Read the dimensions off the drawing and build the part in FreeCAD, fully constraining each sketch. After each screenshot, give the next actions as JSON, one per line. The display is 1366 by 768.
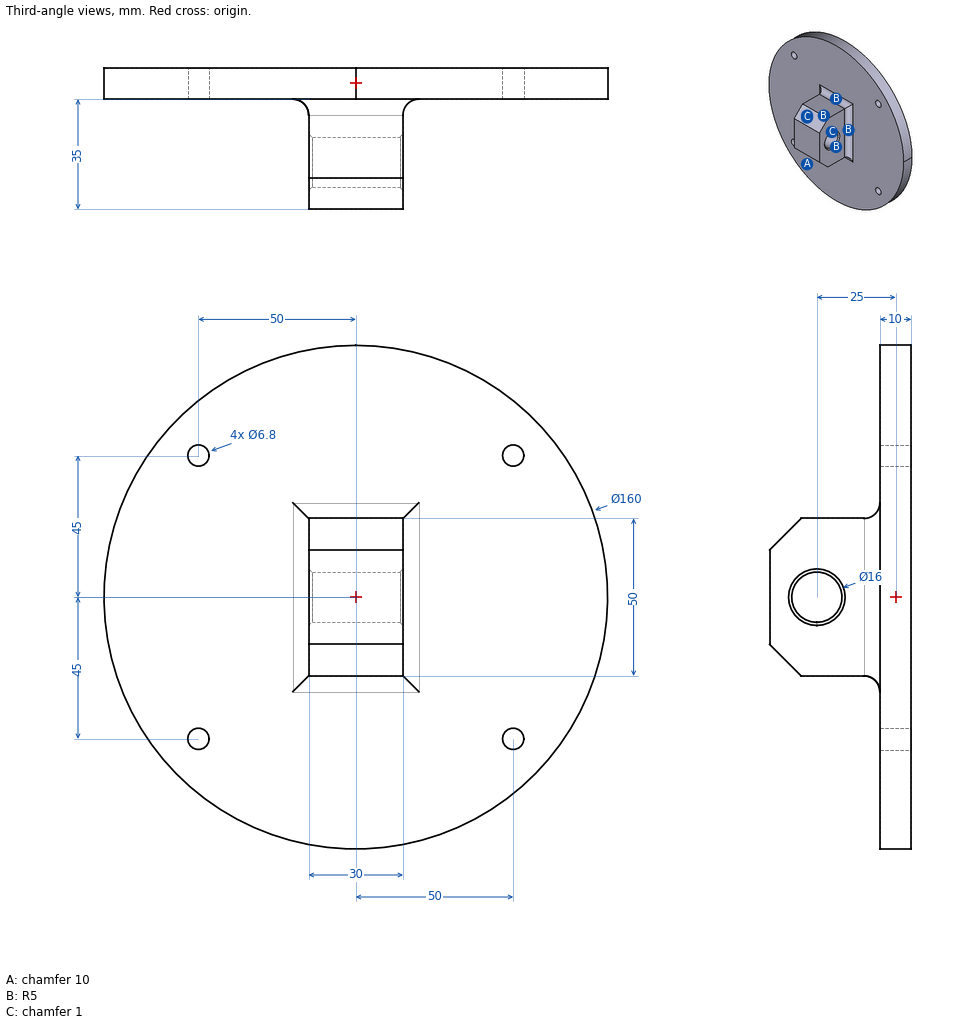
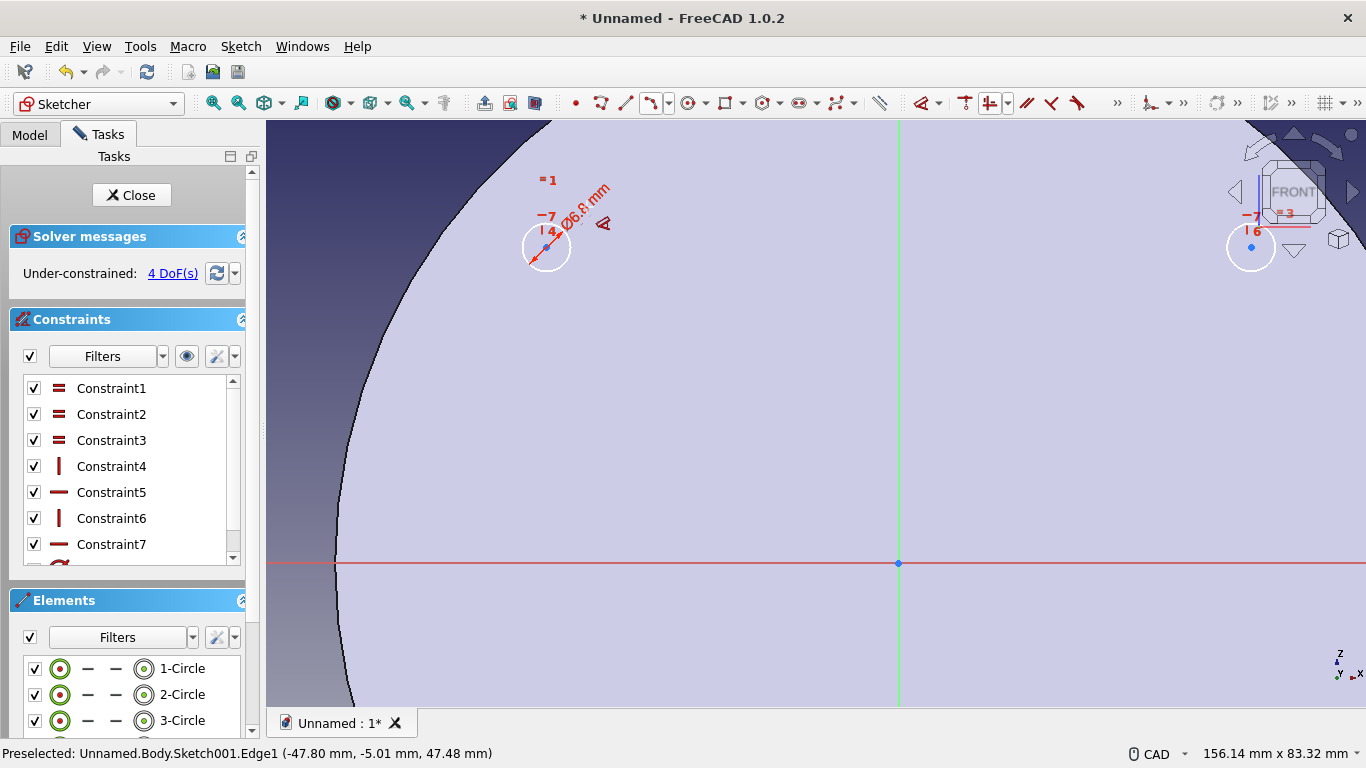
{"action": "left_click", "coordinate": [547, 247]}
{"action": "left_click", "coordinate": [723, 213]}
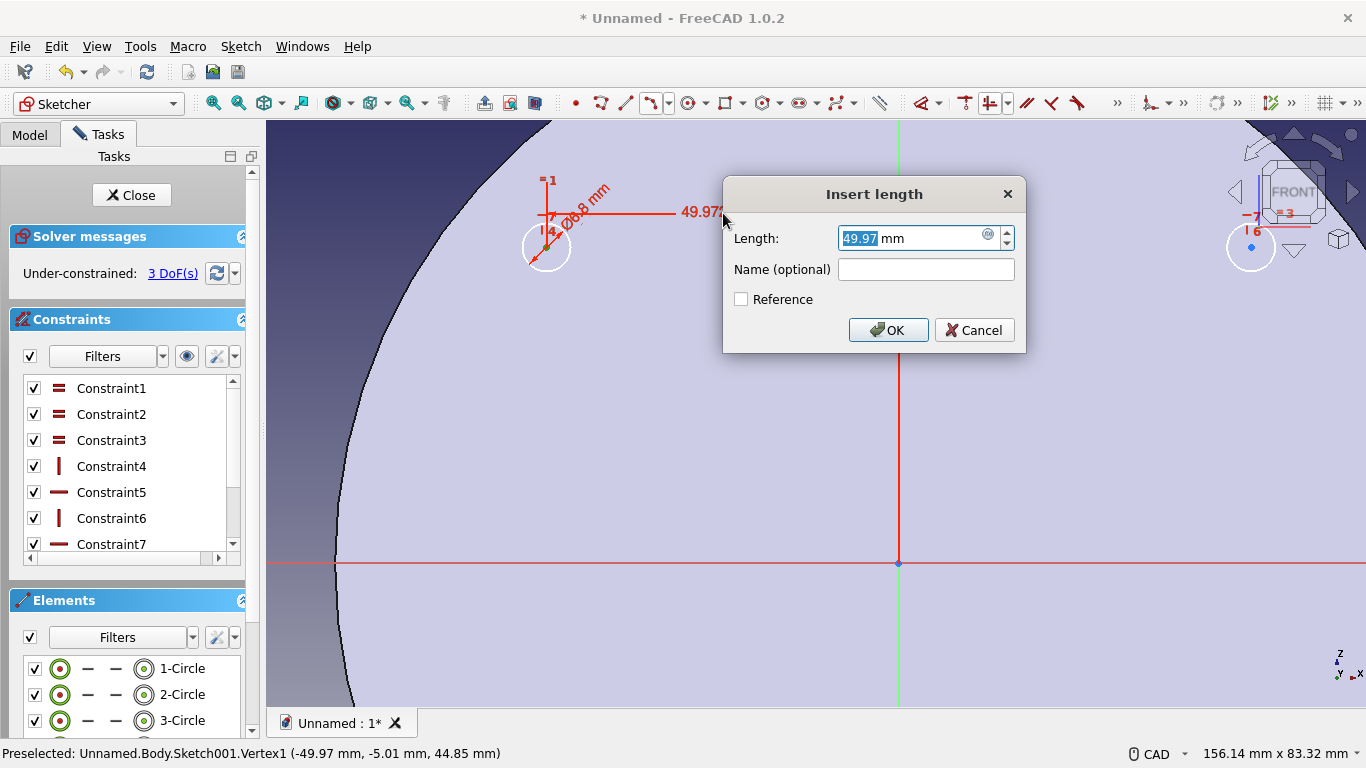
{"action": "type", "text": "50"}
{"action": "key", "text": "Return"}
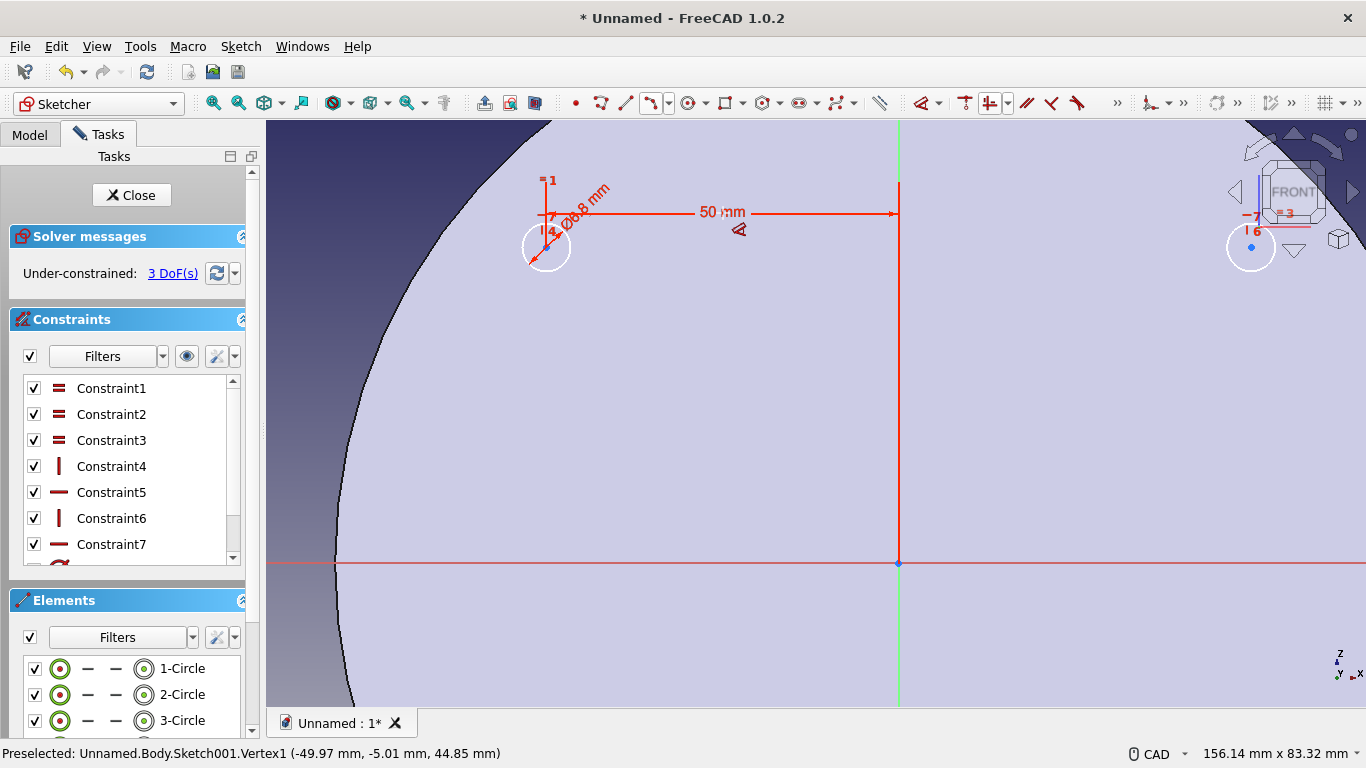
{"action": "left_click", "coordinate": [546, 247]}
{"action": "left_click", "coordinate": [512, 405]}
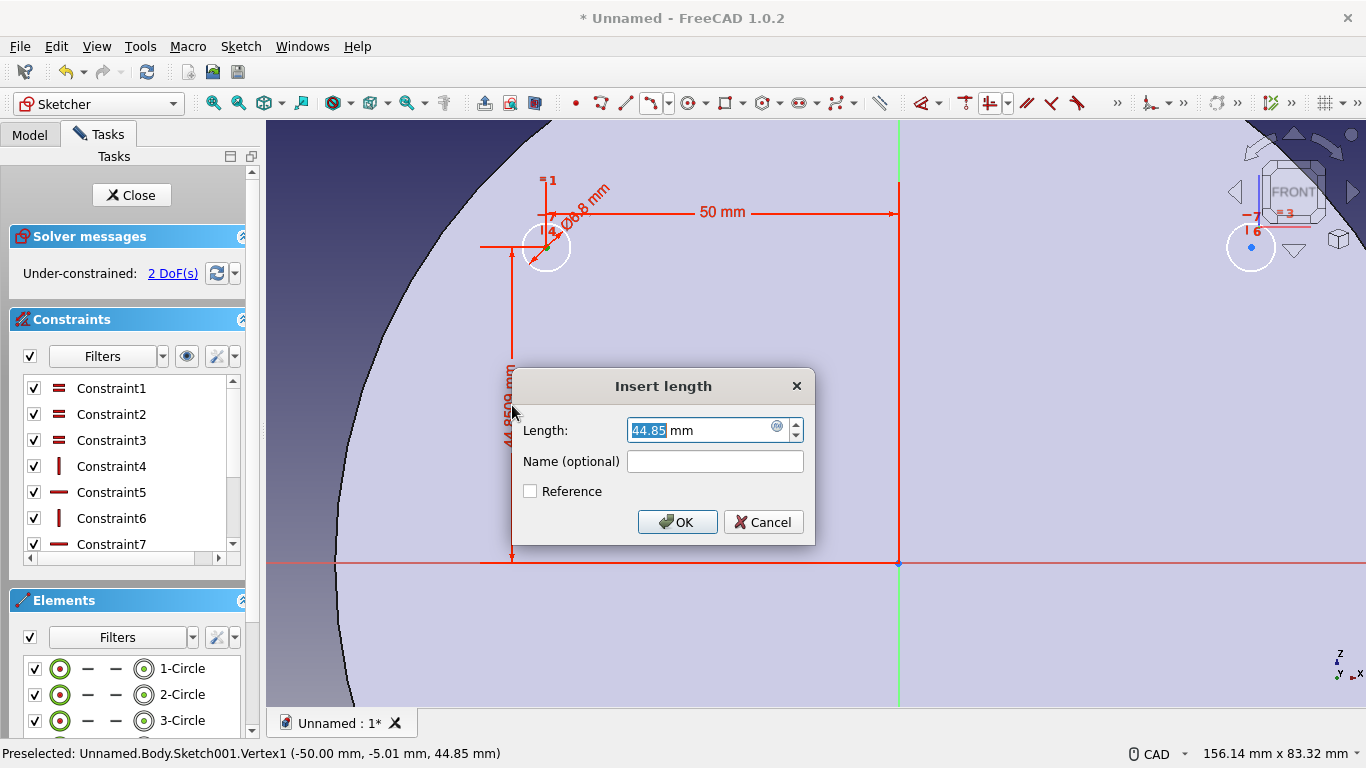
{"action": "type", "text": "45"}
{"action": "key", "text": "Return"}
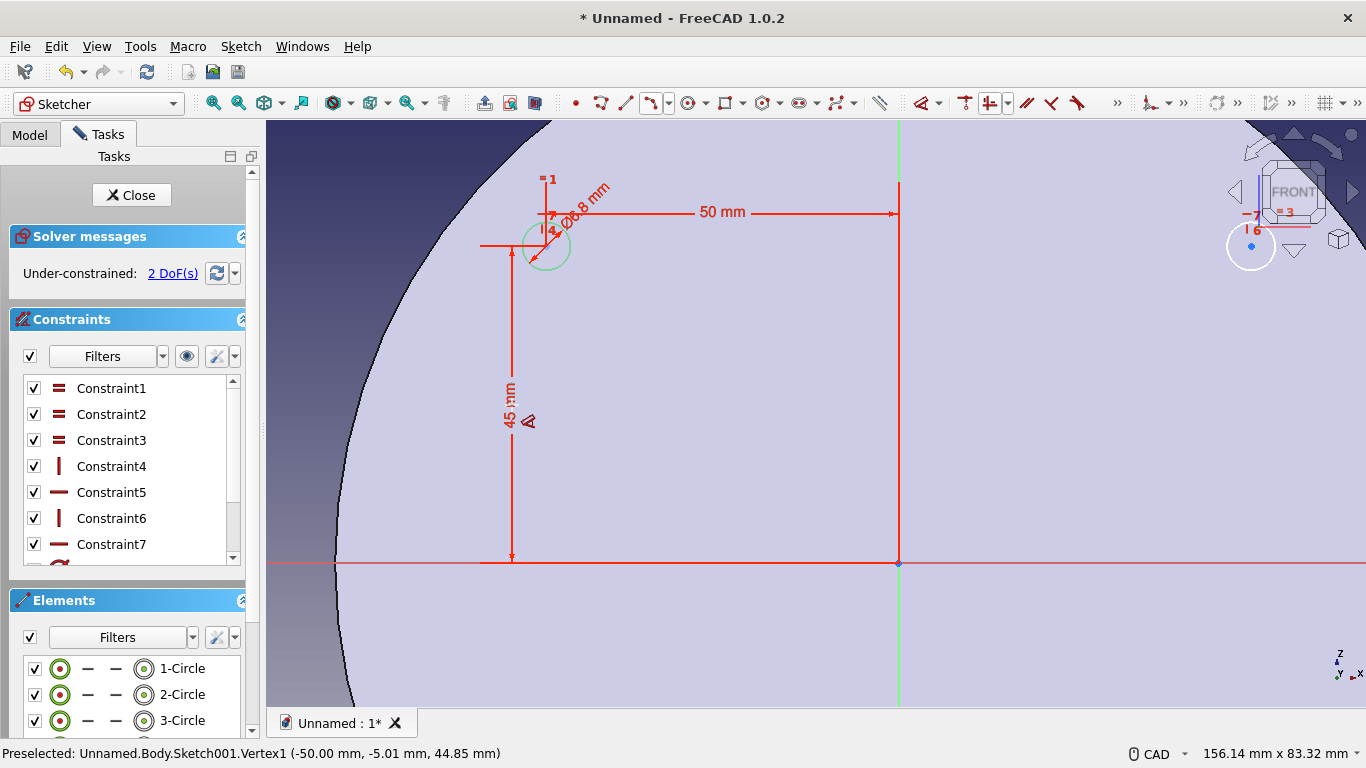
{"action": "scroll", "coordinate": [564, 231], "scroll_direction": "down", "scroll_amount": 3}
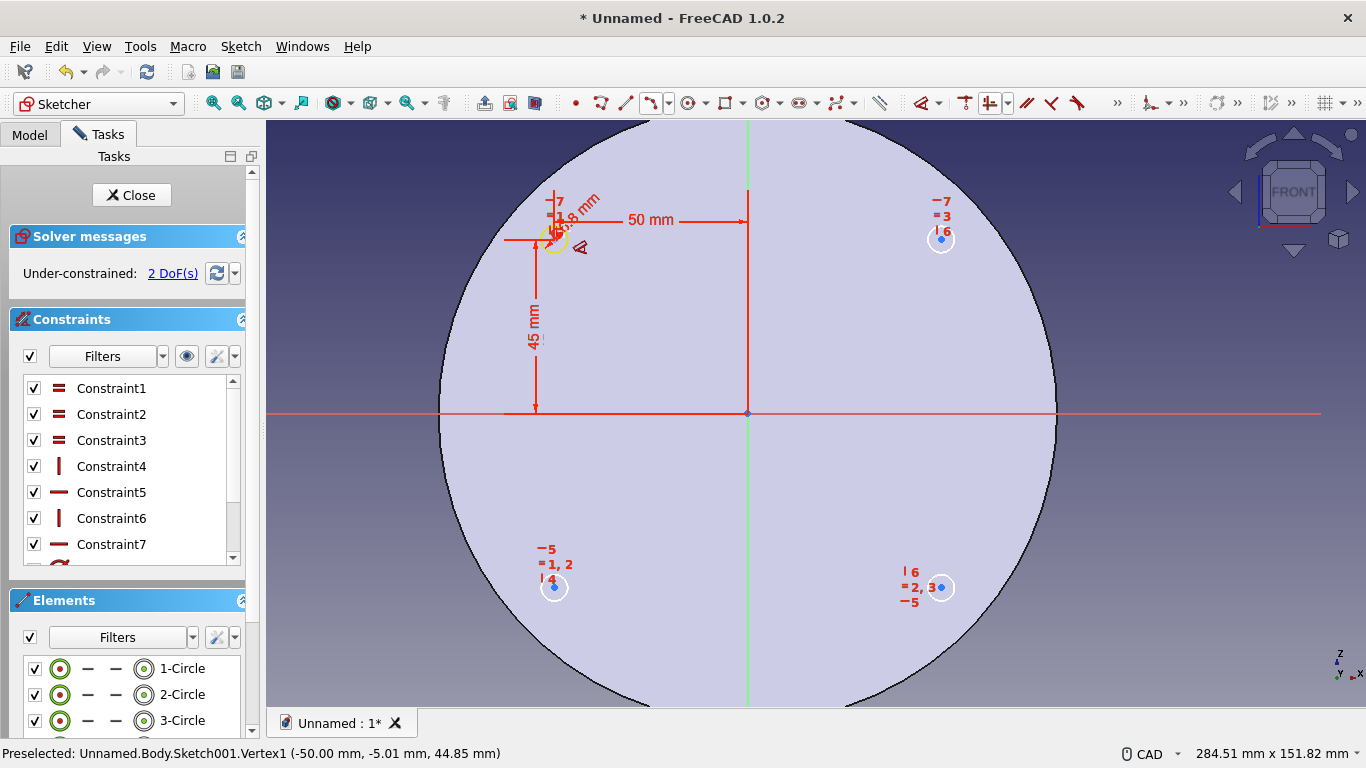
{"action": "left_click", "coordinate": [554, 588]}
{"action": "left_click", "coordinate": [520, 501]}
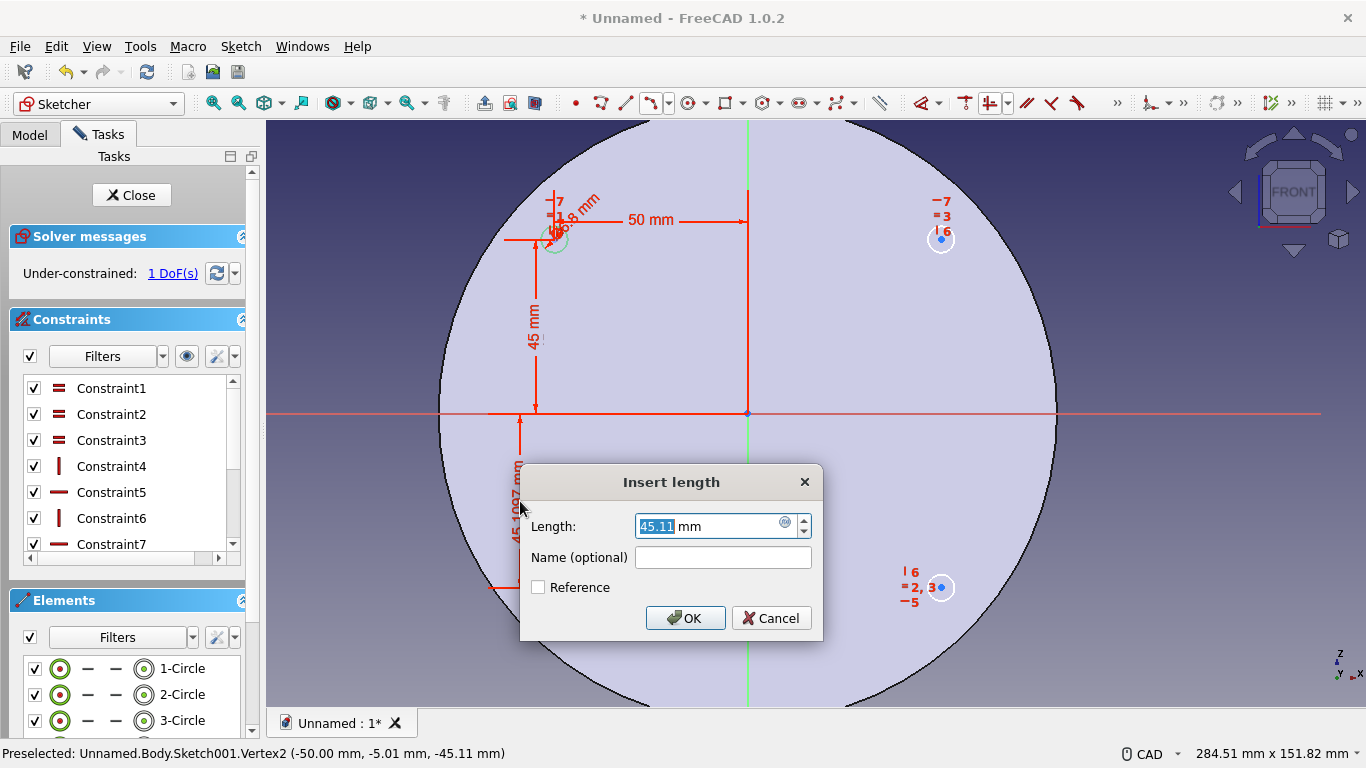
{"action": "type", "text": "45"}
{"action": "key", "text": "Return"}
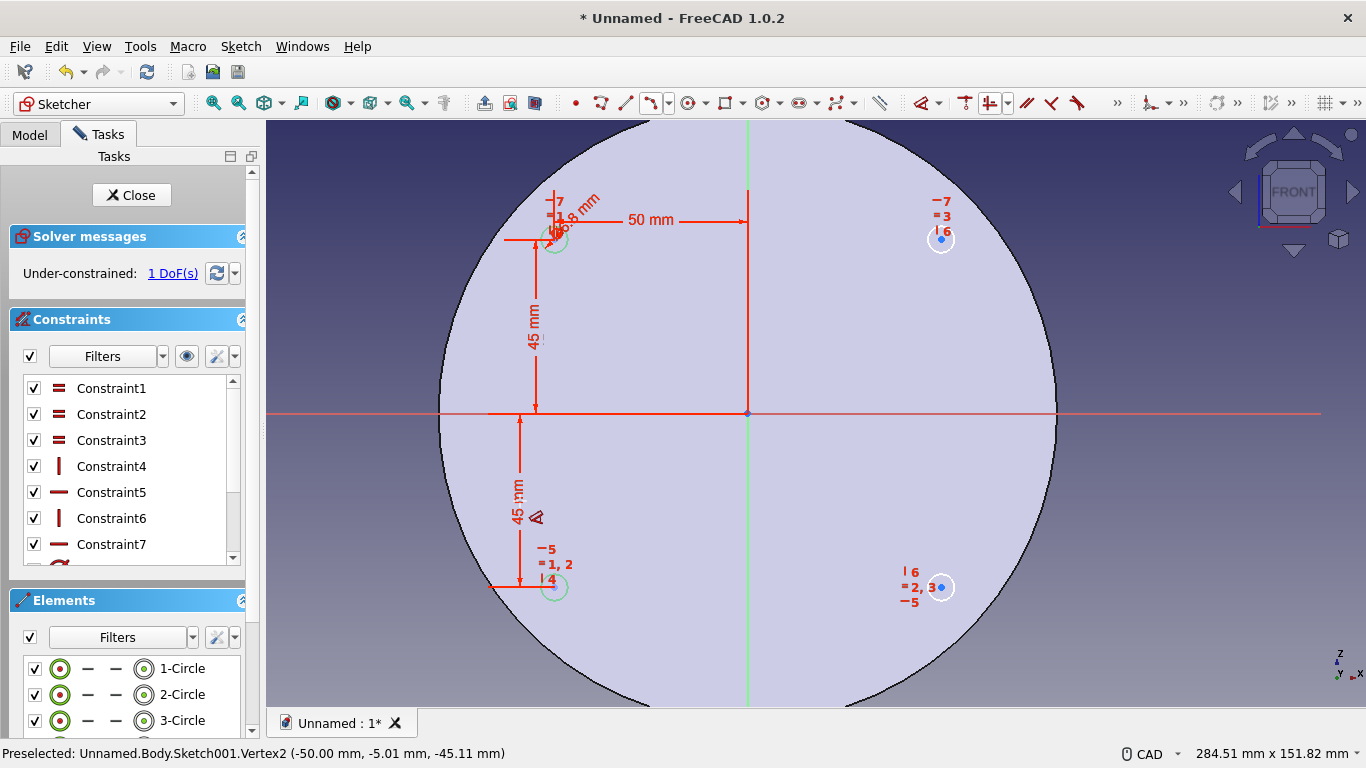
{"action": "left_click", "coordinate": [941, 587]}
{"action": "left_click", "coordinate": [845, 621]}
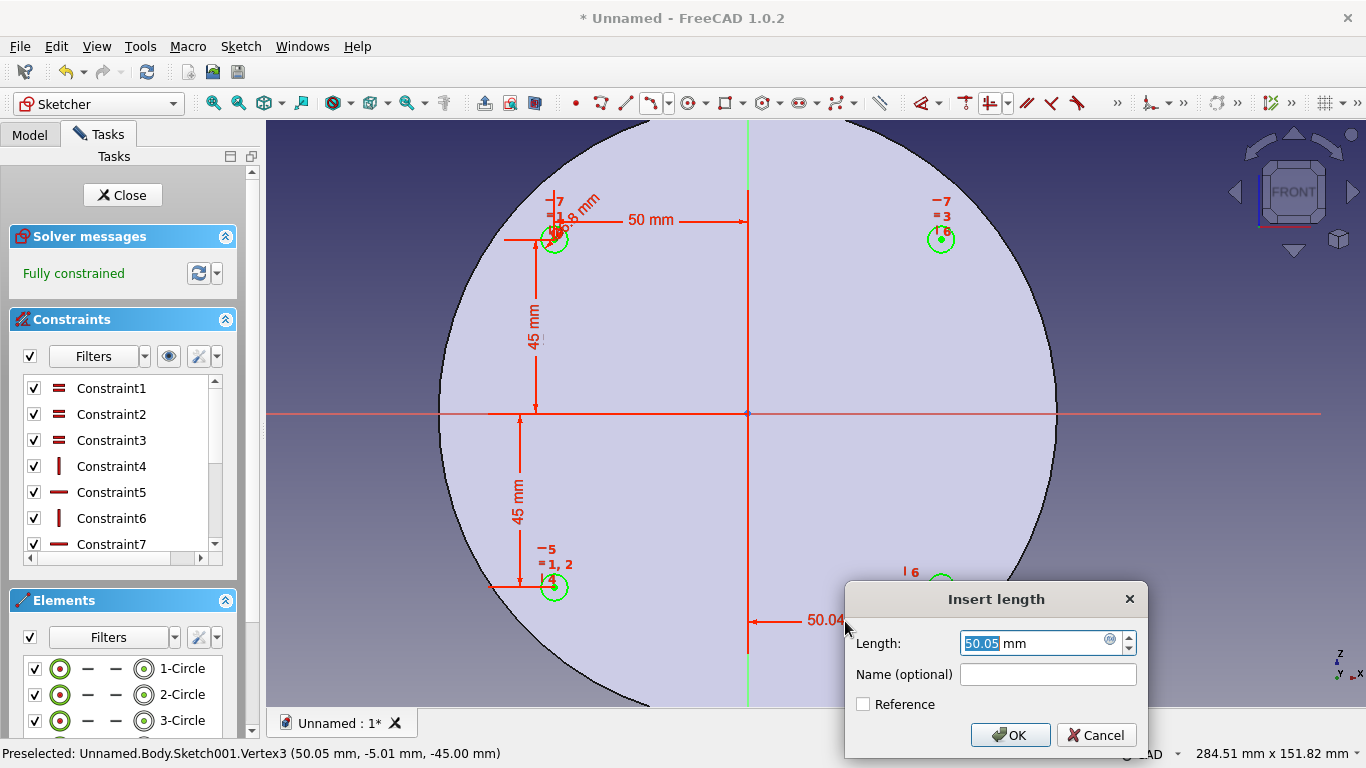
{"action": "type", "text": "50"}
{"action": "key", "text": "Return"}
{"action": "key", "text": "Escape"}